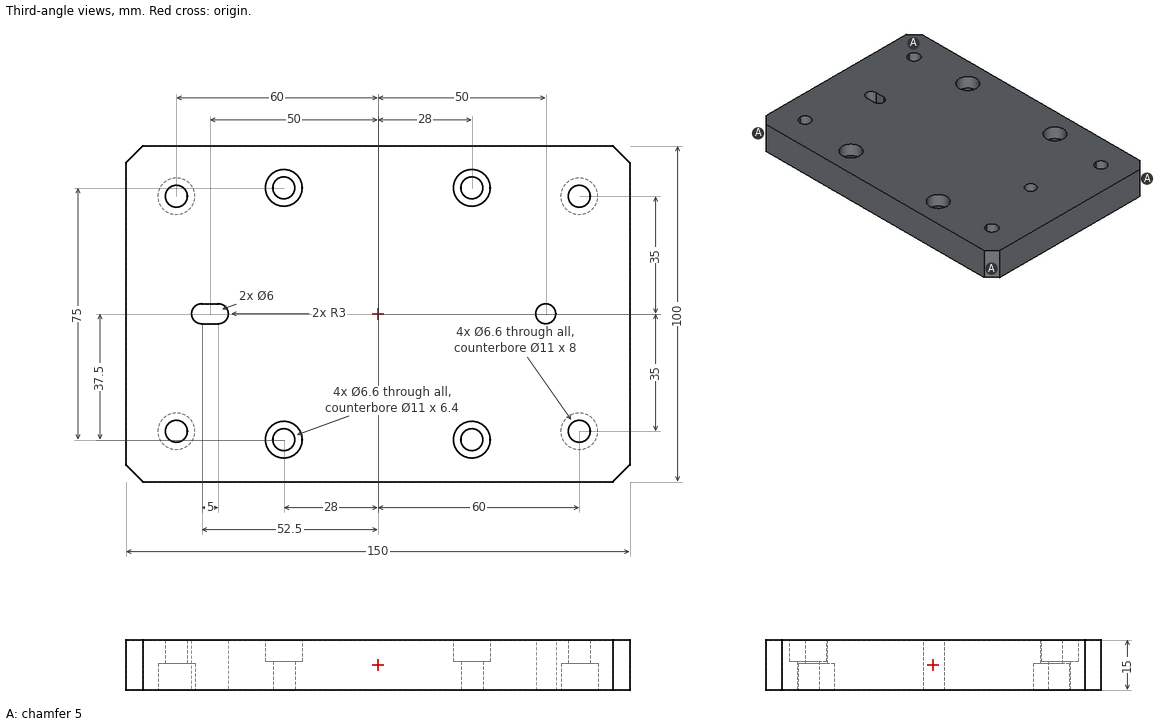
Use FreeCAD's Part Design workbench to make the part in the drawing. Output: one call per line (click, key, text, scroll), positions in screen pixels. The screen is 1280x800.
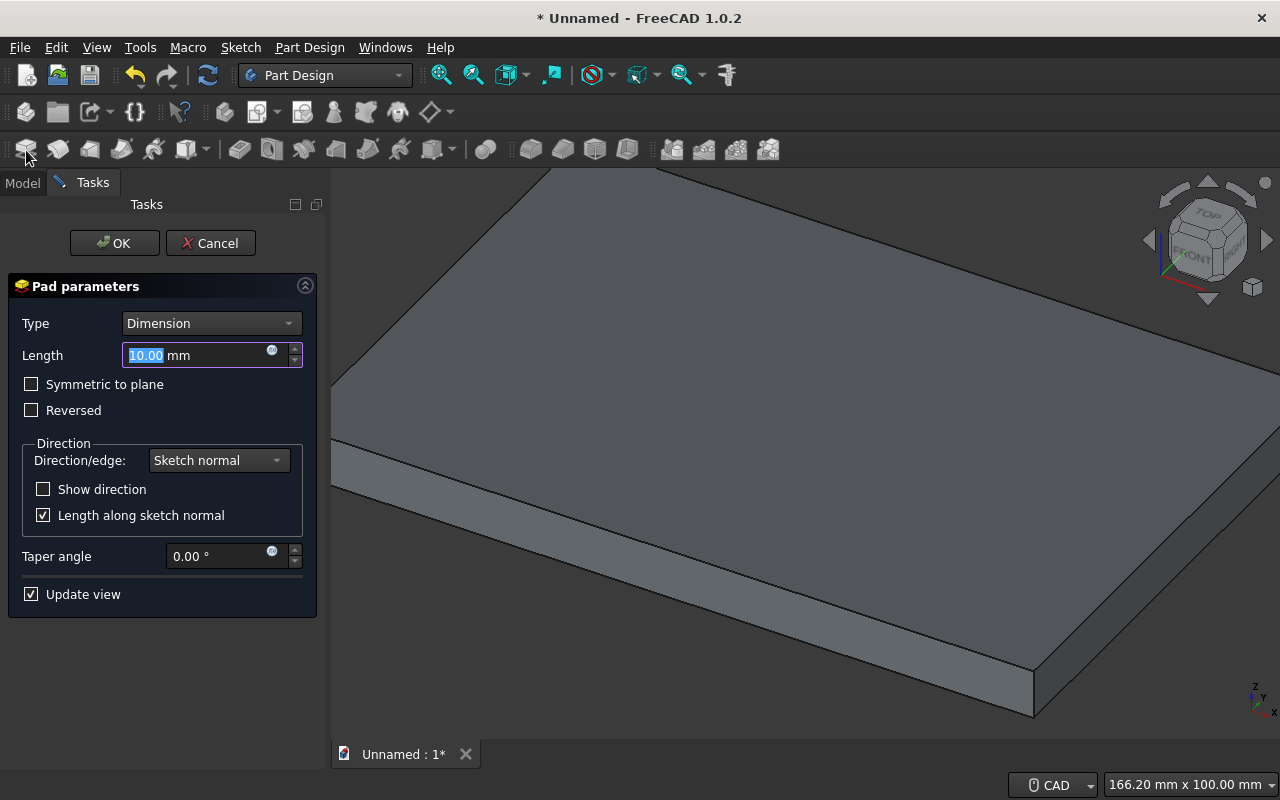
text(15)
key(Tab)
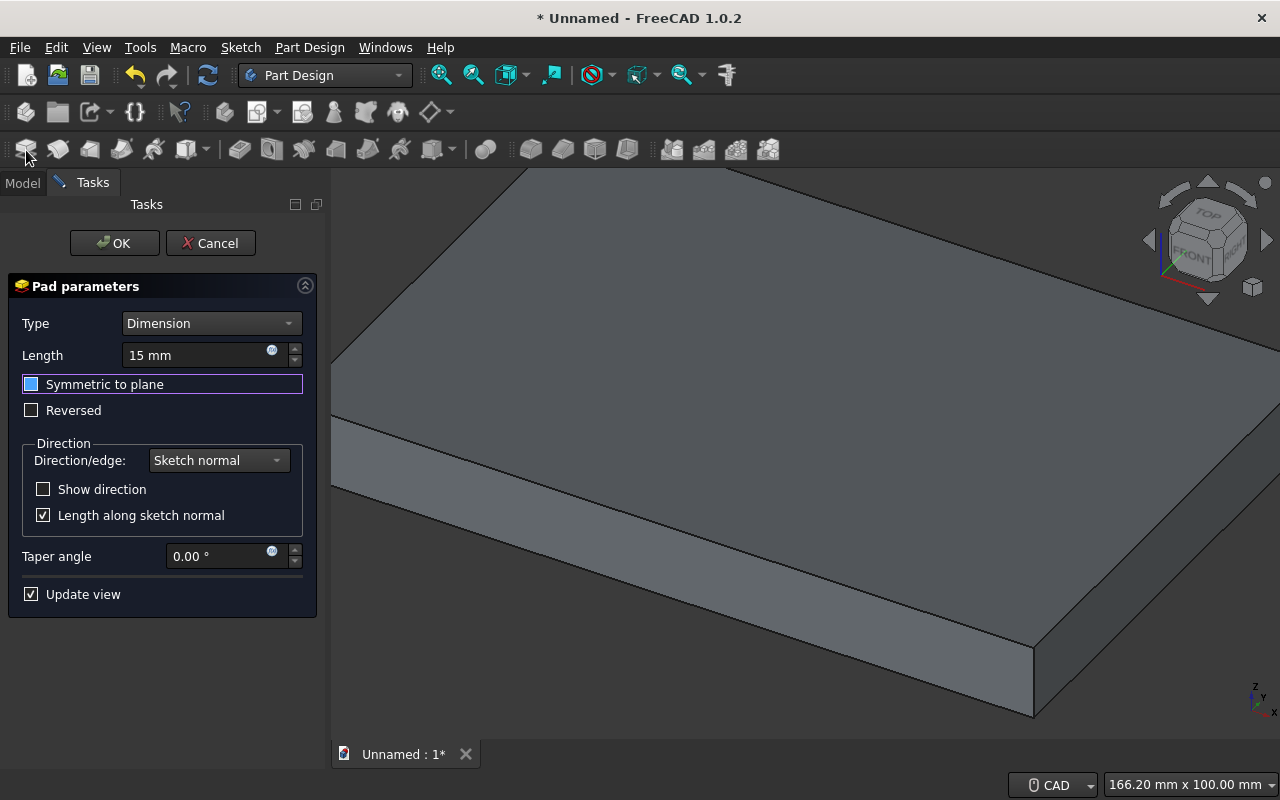
click(30, 384)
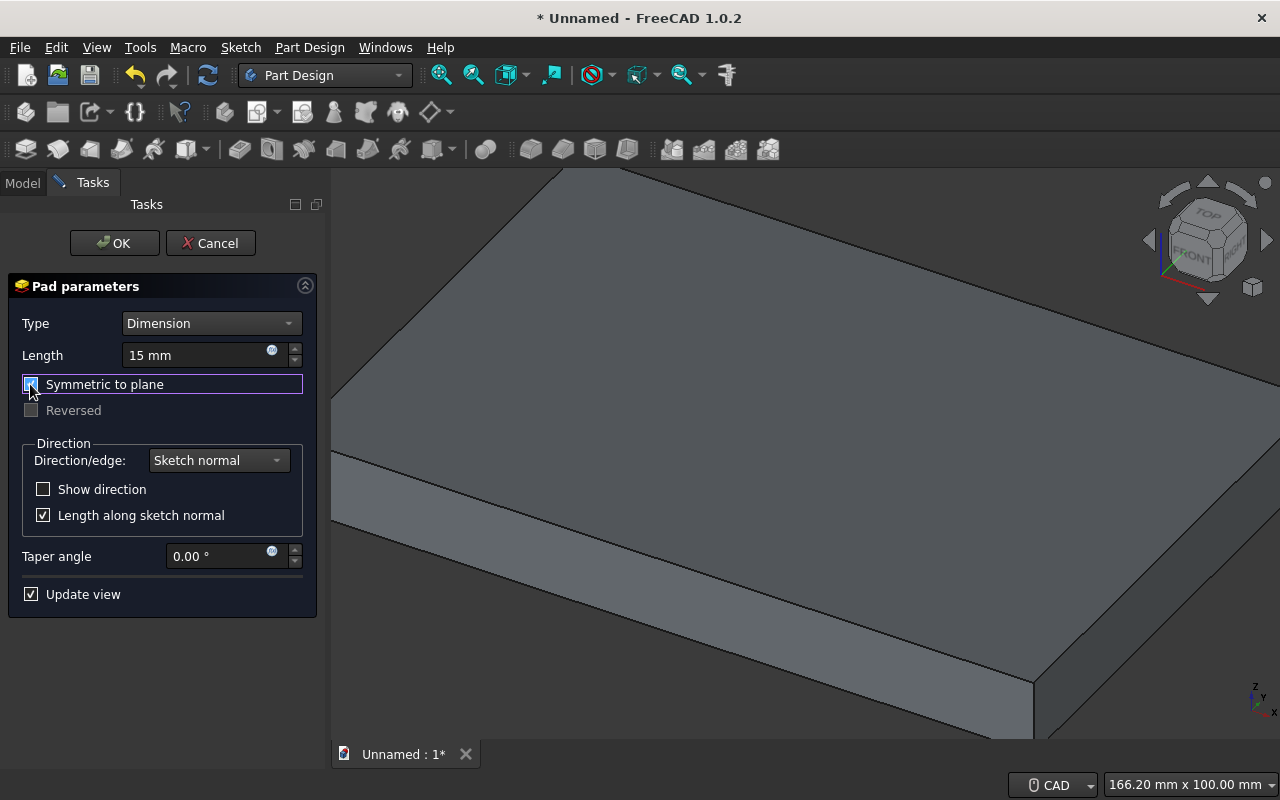
click(115, 243)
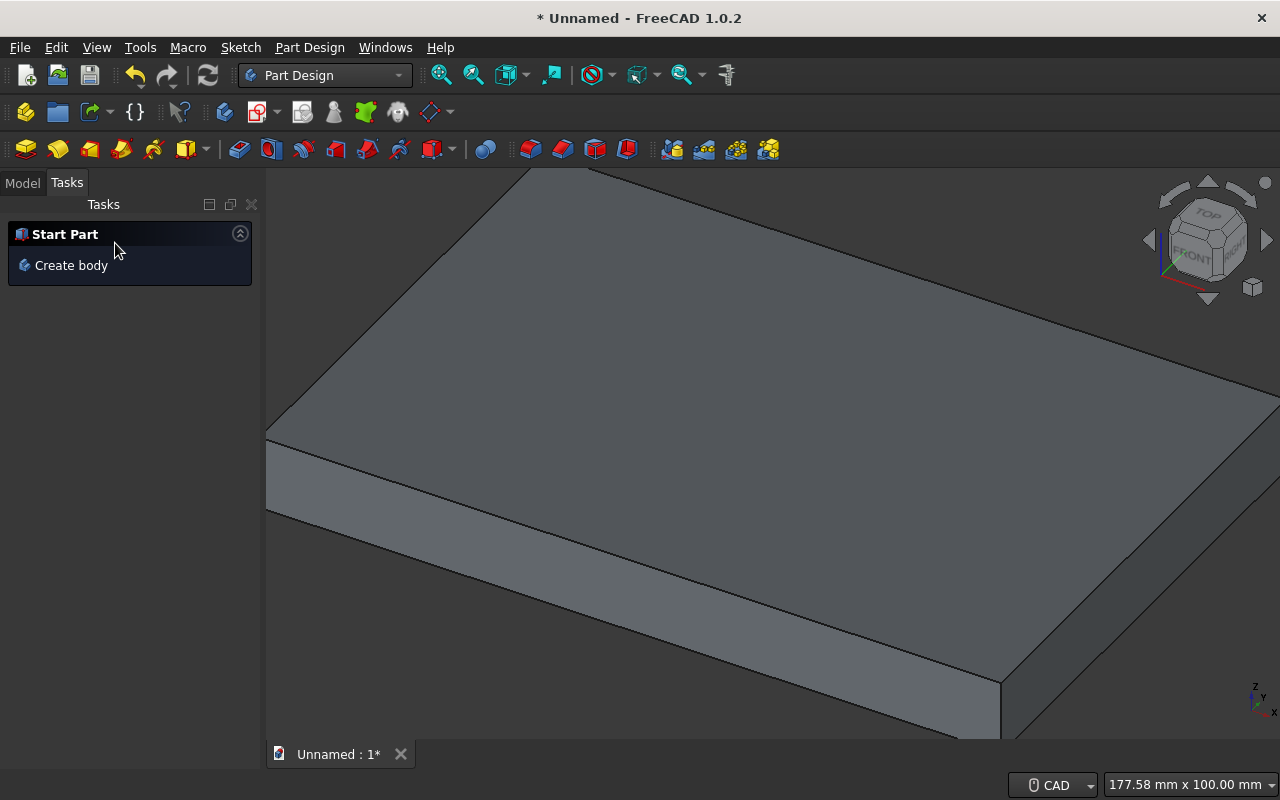
key(v)
key(f)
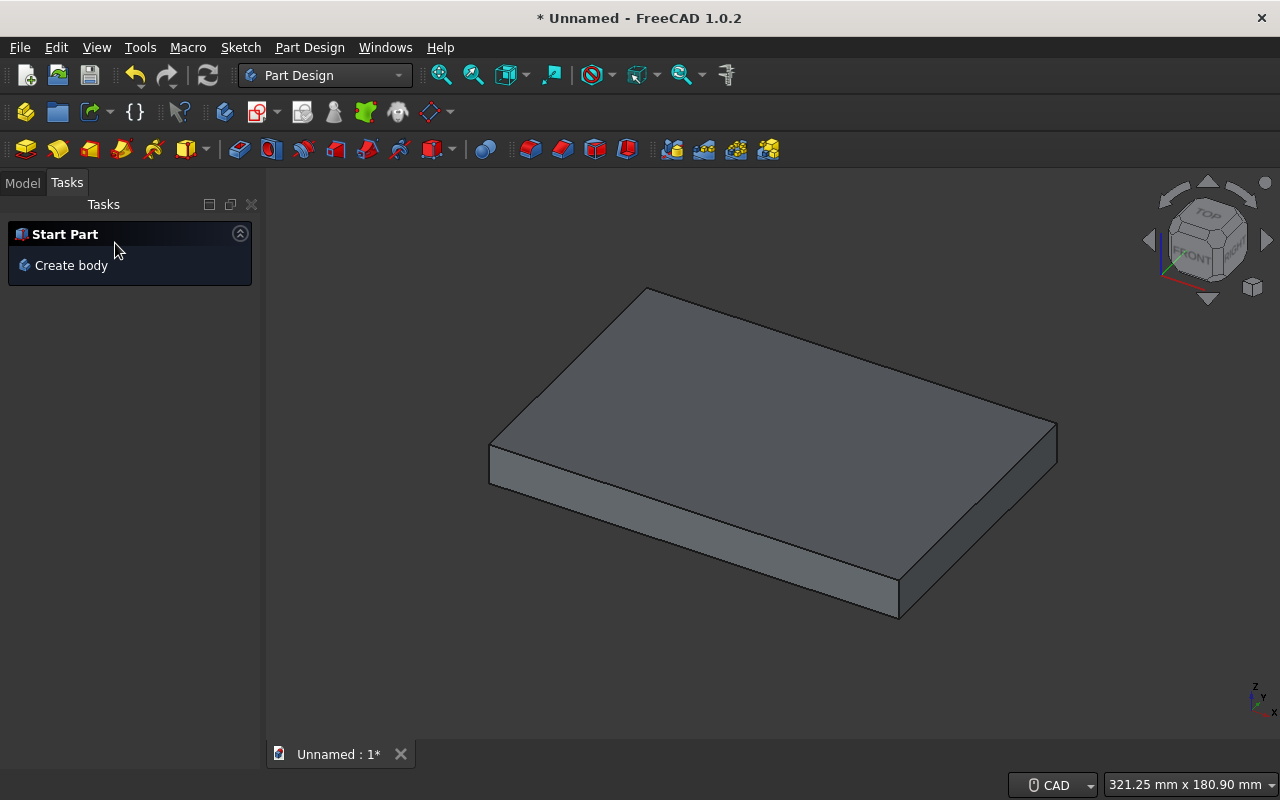
click(832, 453)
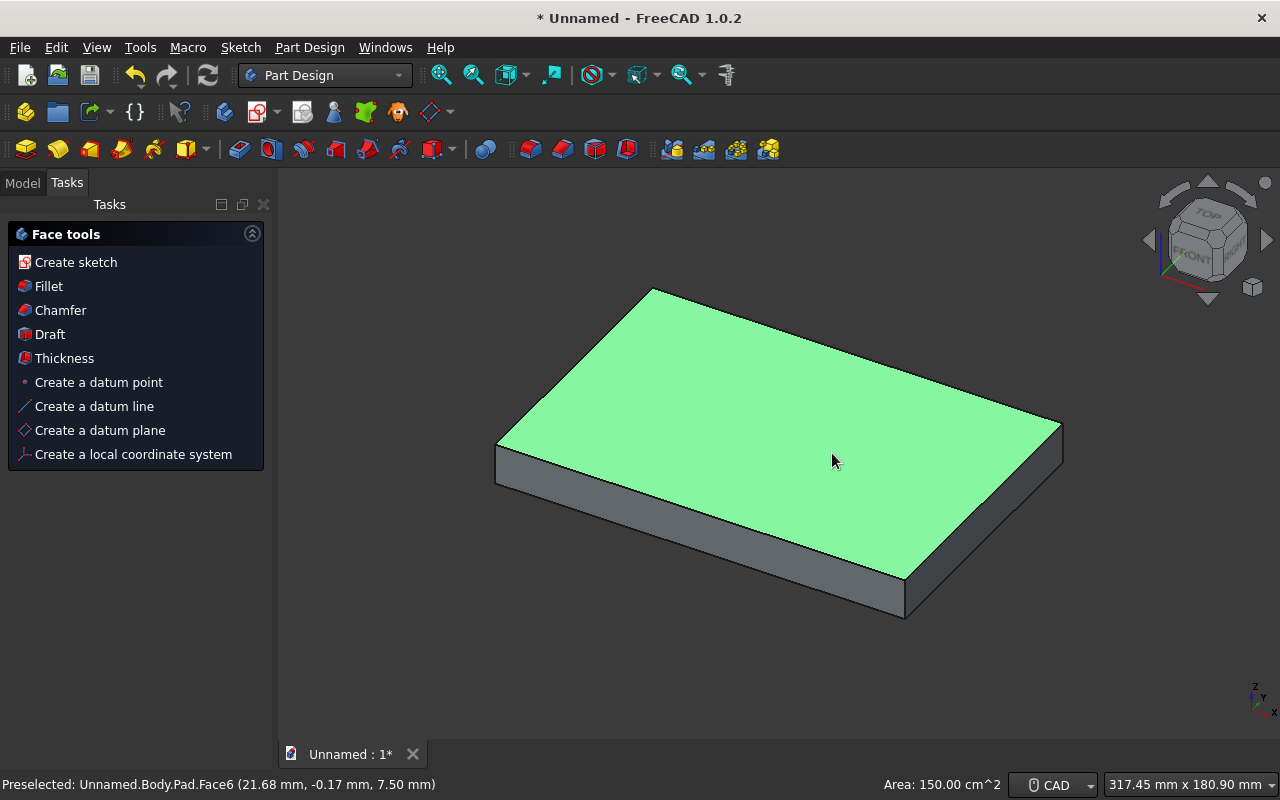
click(258, 112)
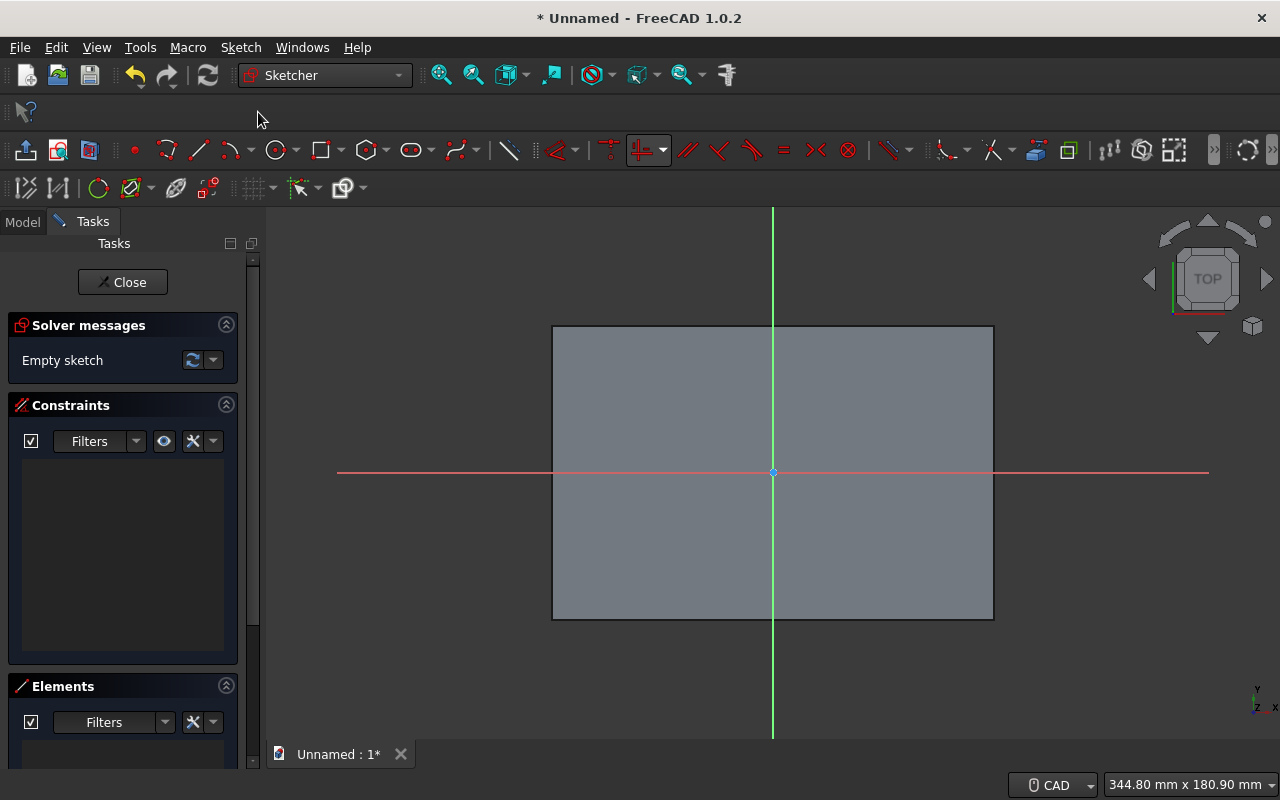
scroll(912, 473, up, 2)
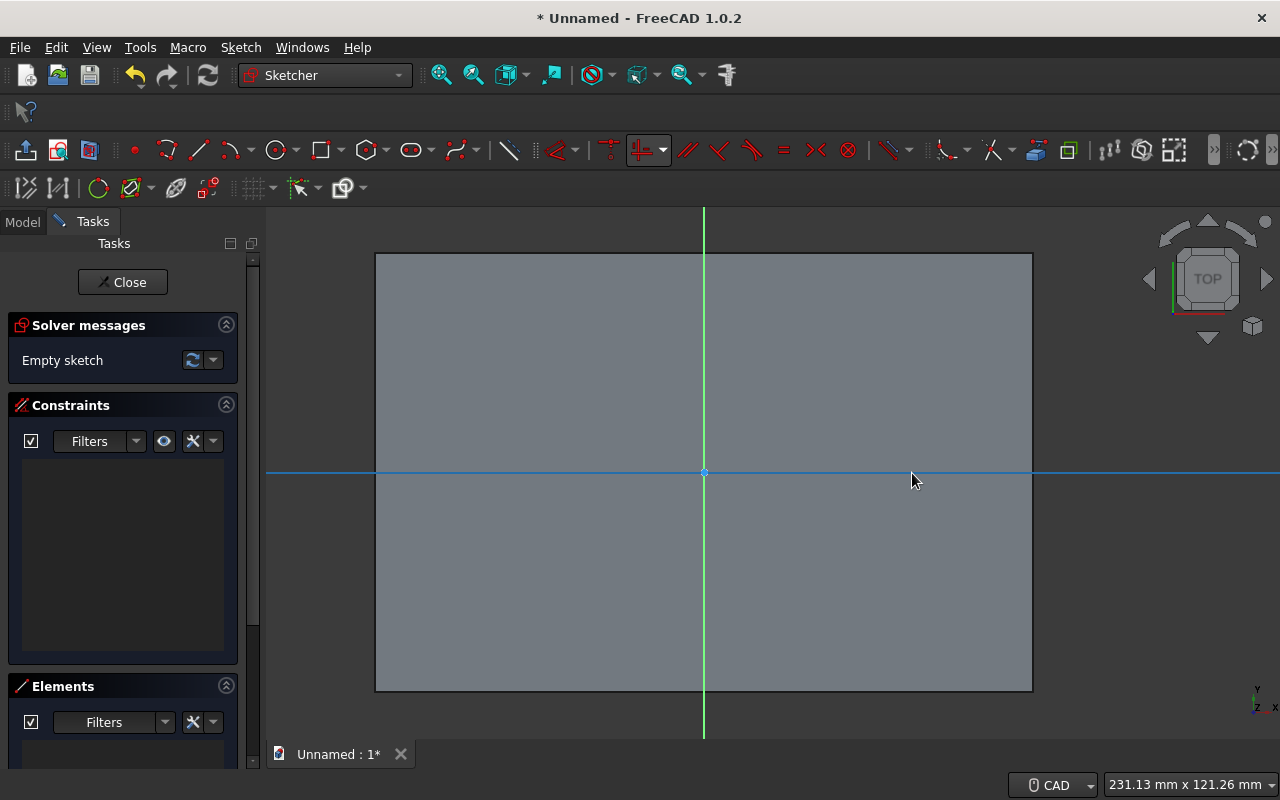
key(g)
key(c)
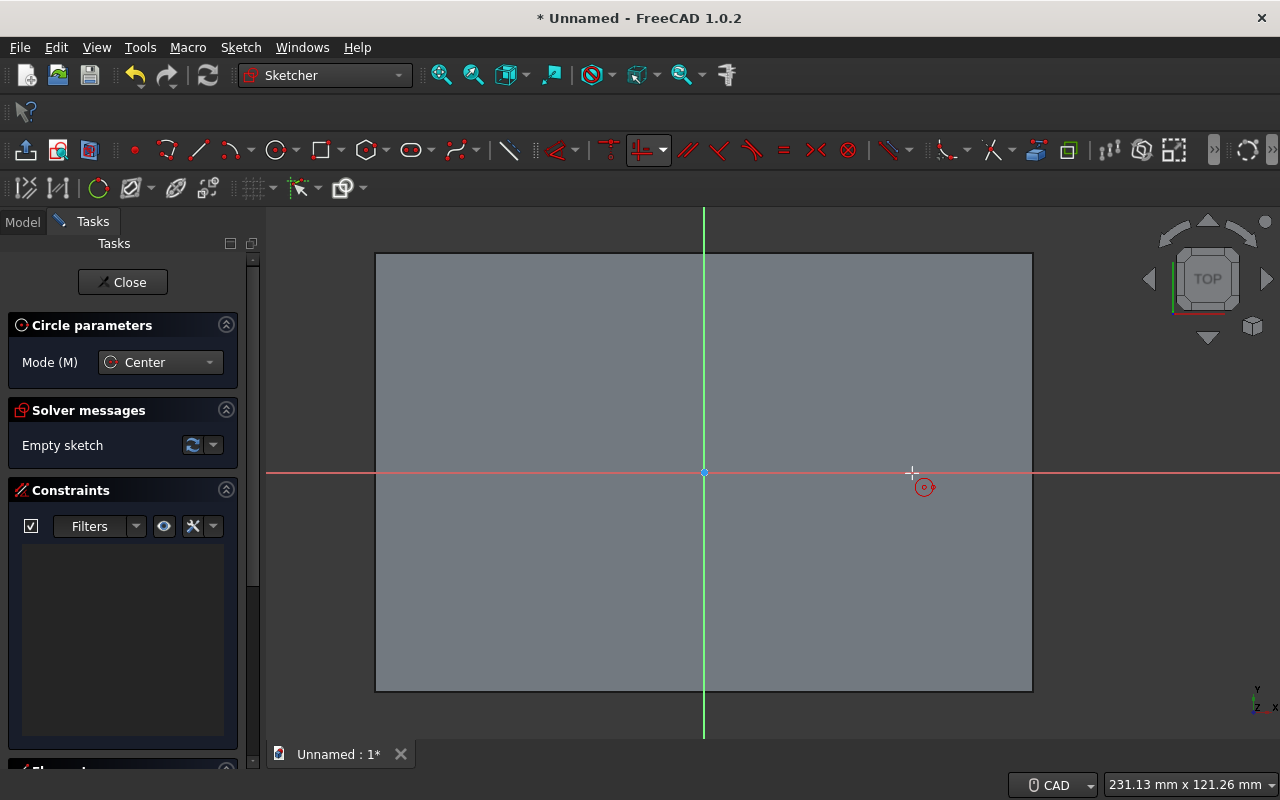
scroll(581, 637, up, 3)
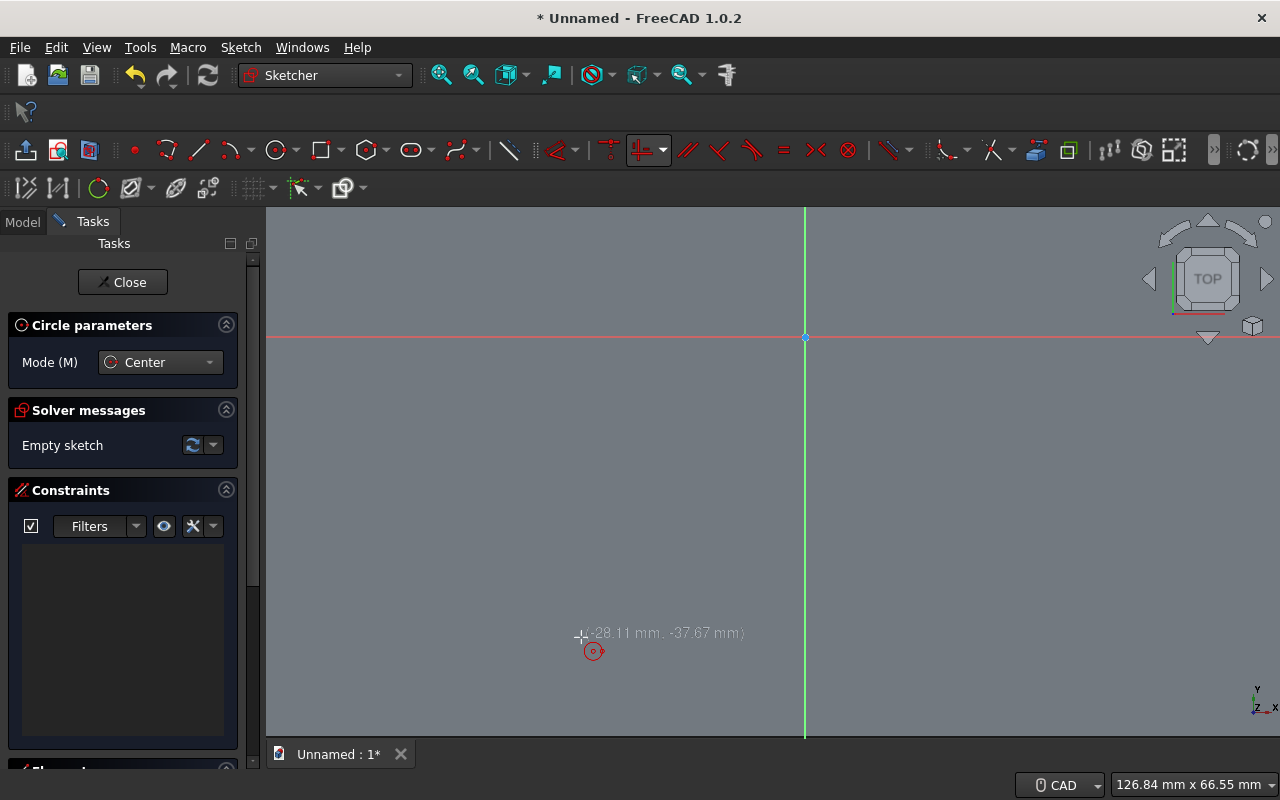
click(582, 637)
move(600, 618)